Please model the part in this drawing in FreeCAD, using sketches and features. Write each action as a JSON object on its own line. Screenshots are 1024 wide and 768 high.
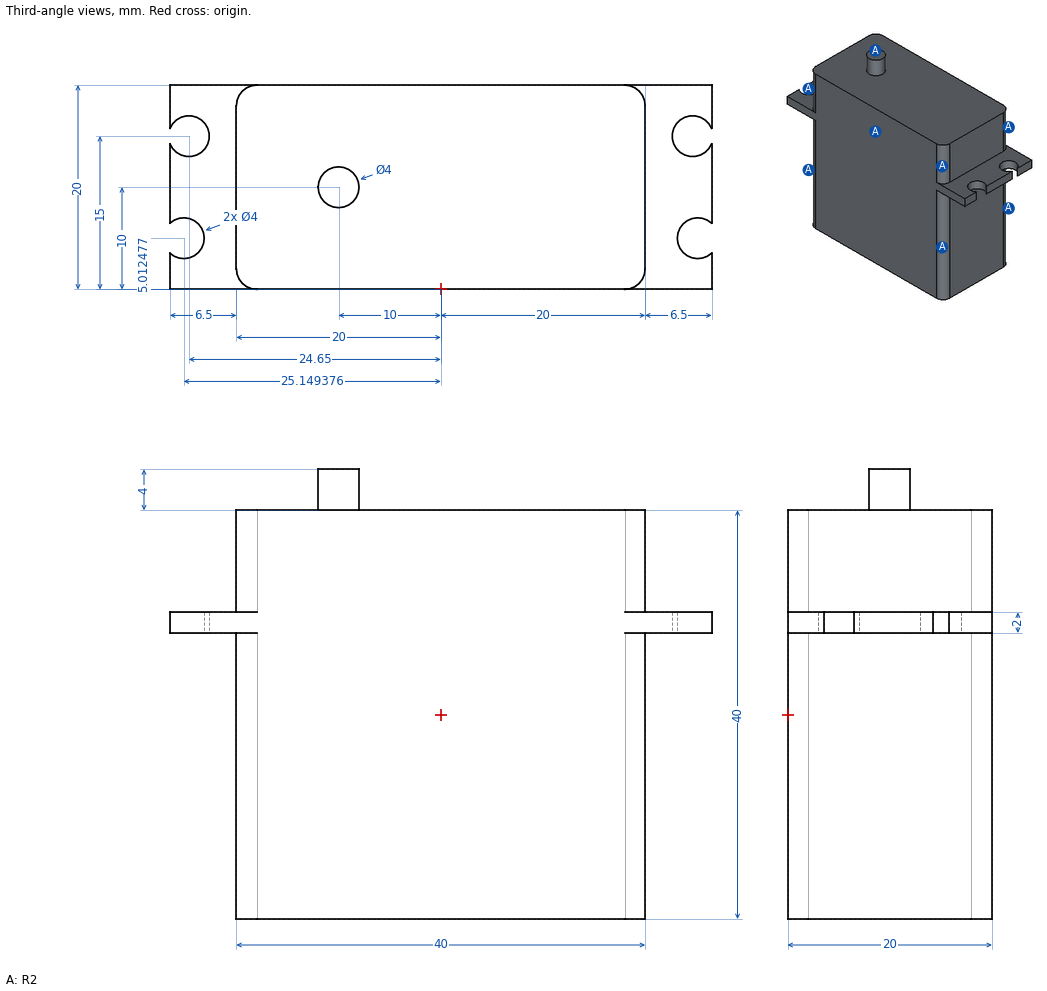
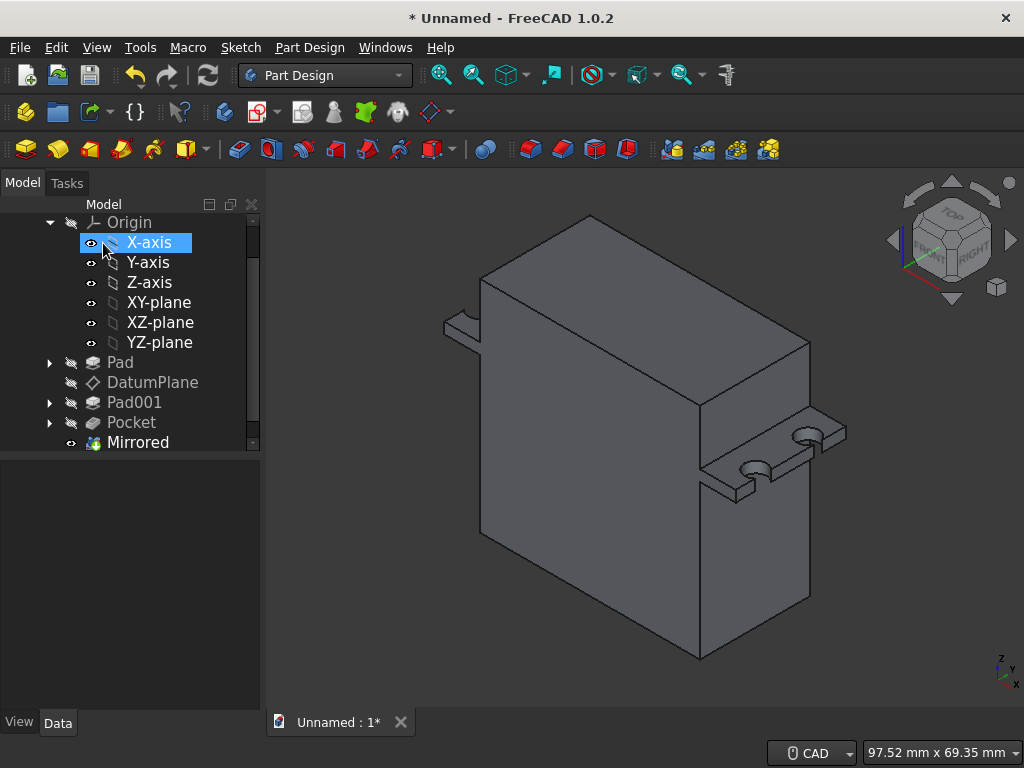
{"action": "left_click", "coordinate": [676, 328]}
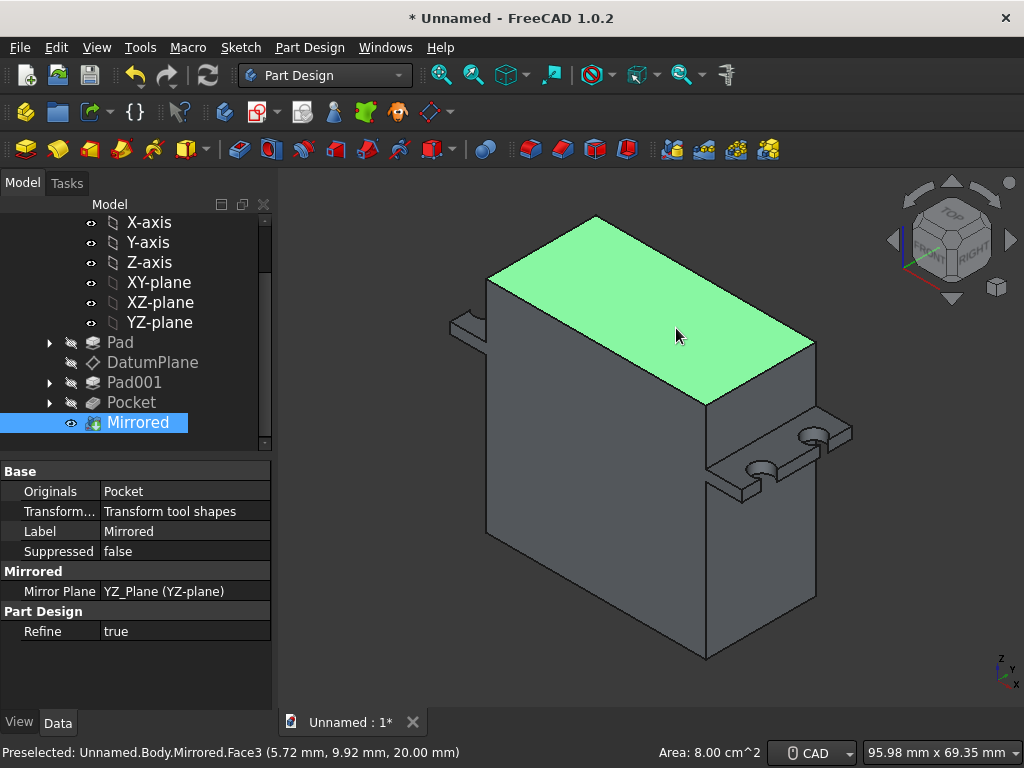
{"action": "left_click", "coordinate": [258, 112]}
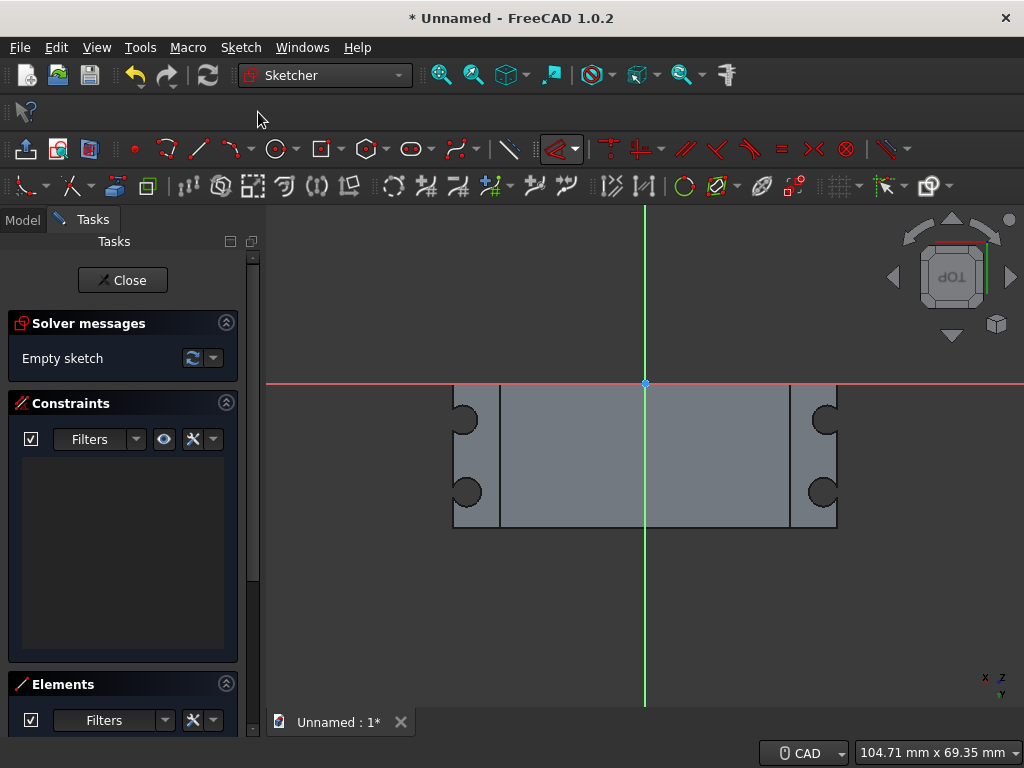
{"action": "scroll", "coordinate": [731, 456], "scroll_direction": "up", "scroll_amount": 12}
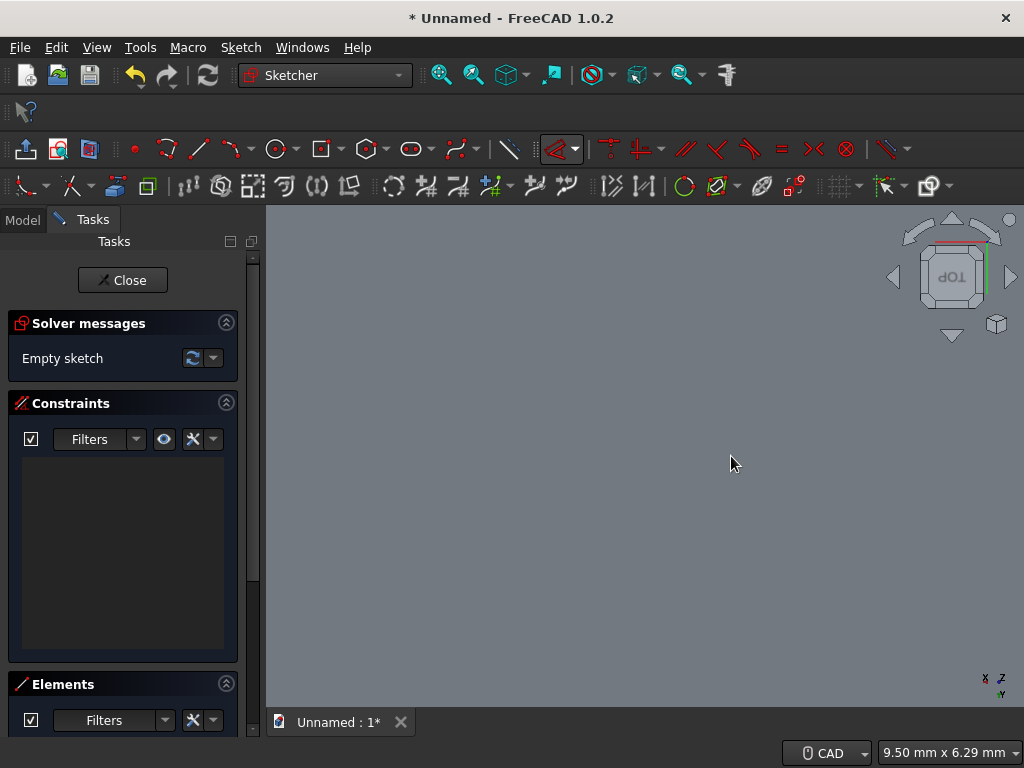
{"action": "left_click", "coordinate": [276, 150]}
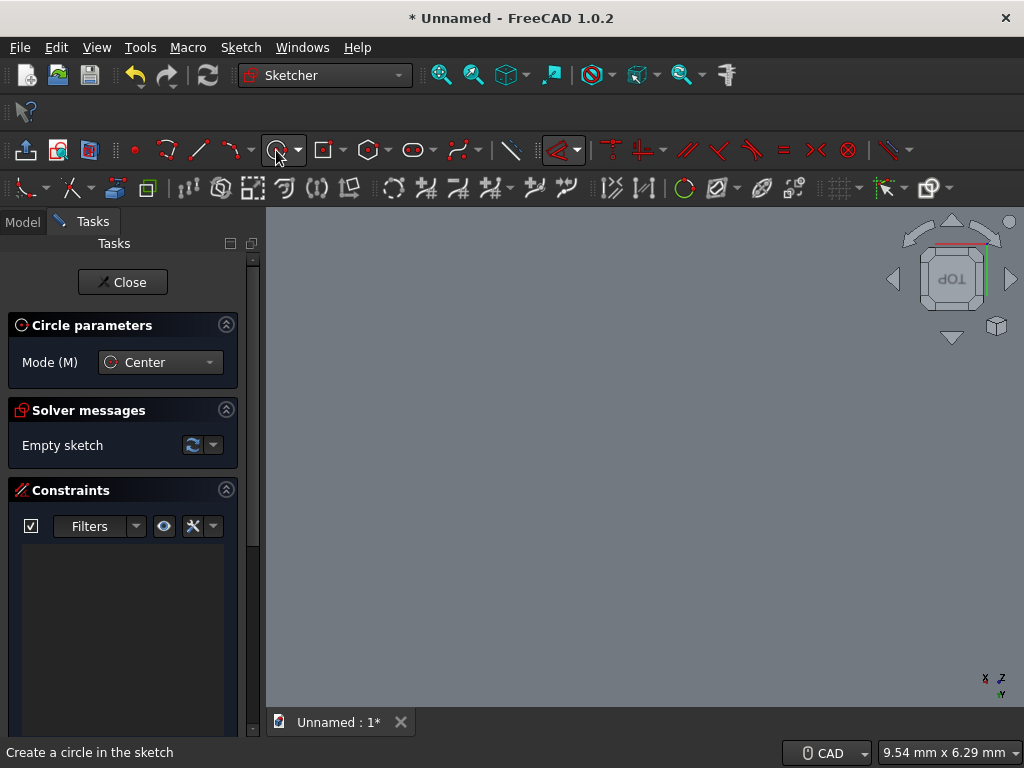
{"action": "left_click", "coordinate": [575, 452]}
{"action": "left_click", "coordinate": [687, 340]}
{"action": "key", "text": "Escape"}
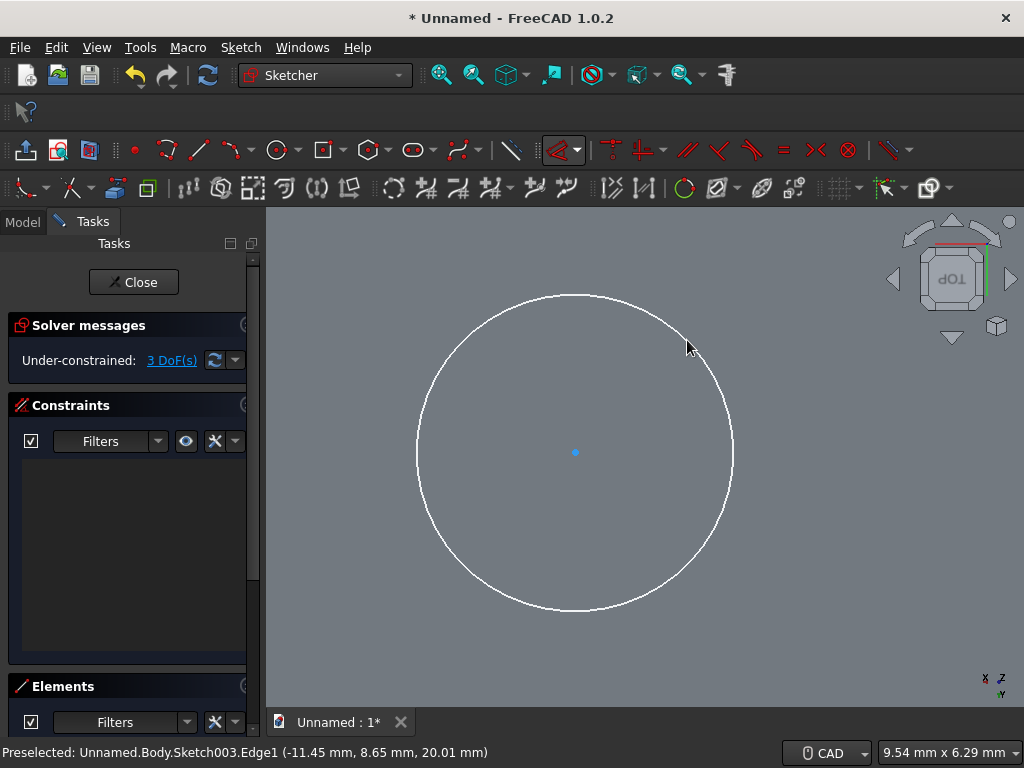
{"action": "left_click", "coordinate": [687, 341]}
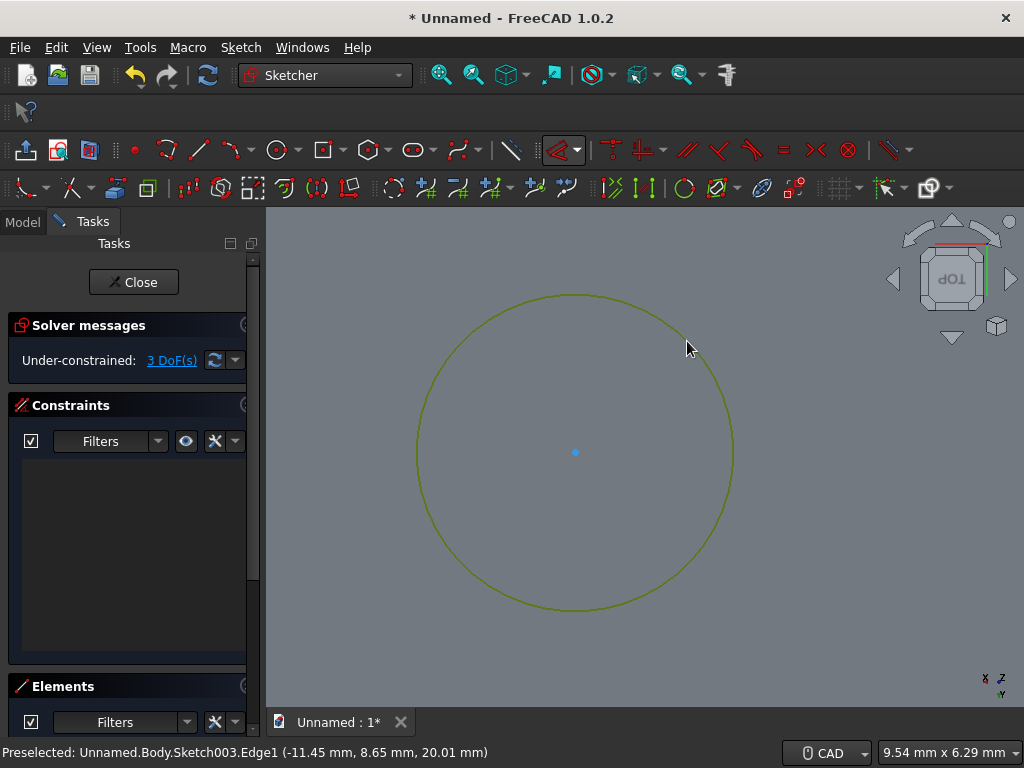
{"action": "key", "text": "k o"}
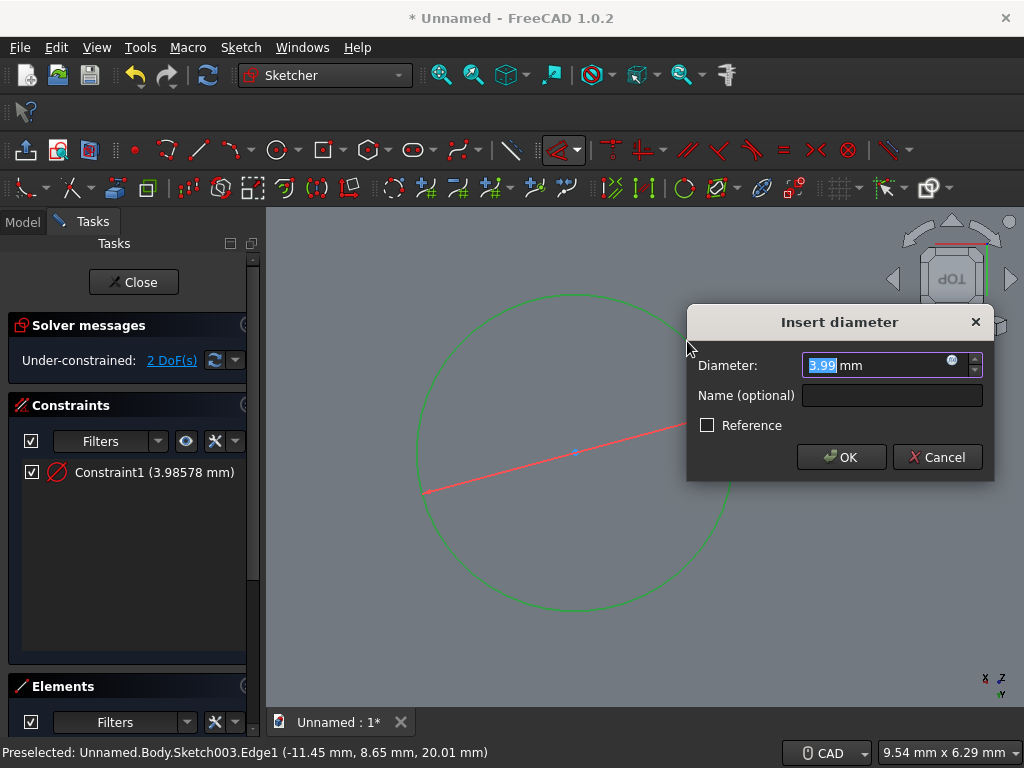
{"action": "type", "text": "4"}
{"action": "key", "text": "Return"}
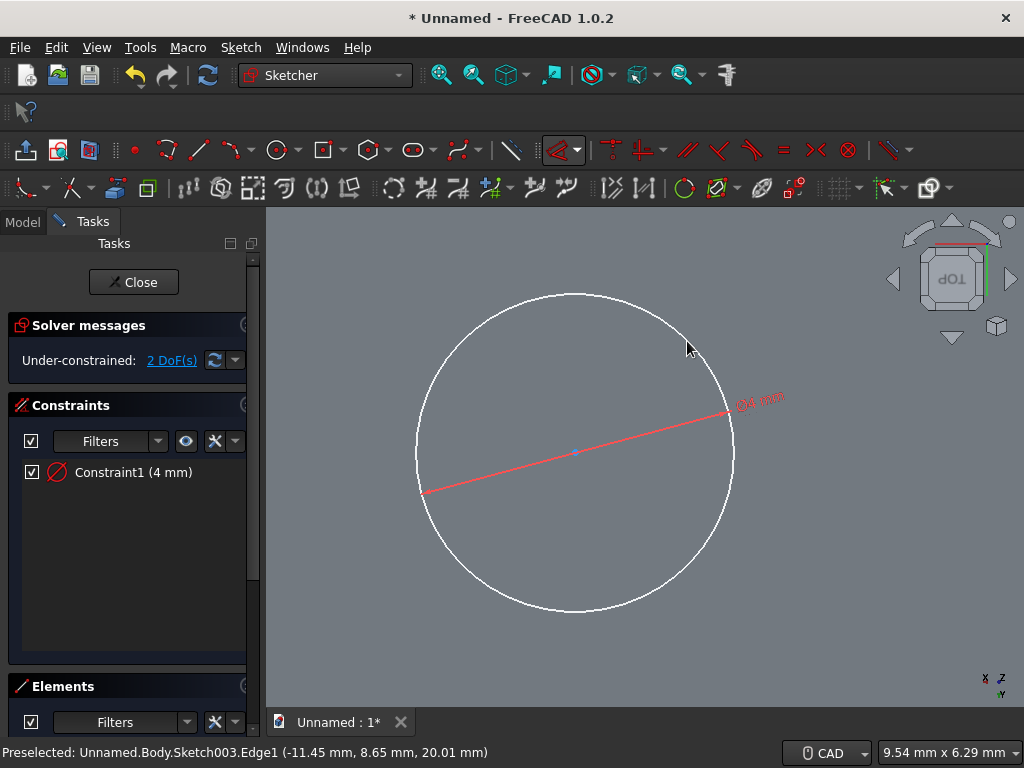
{"action": "left_click", "coordinate": [575, 453]}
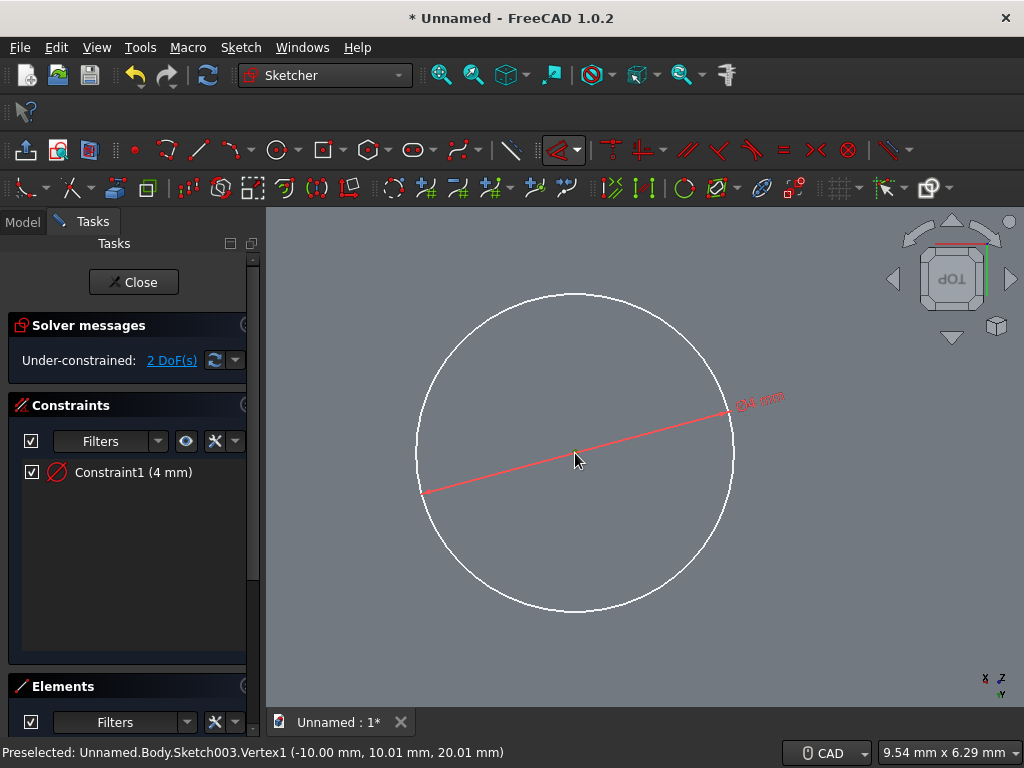
{"action": "key", "text": "l"}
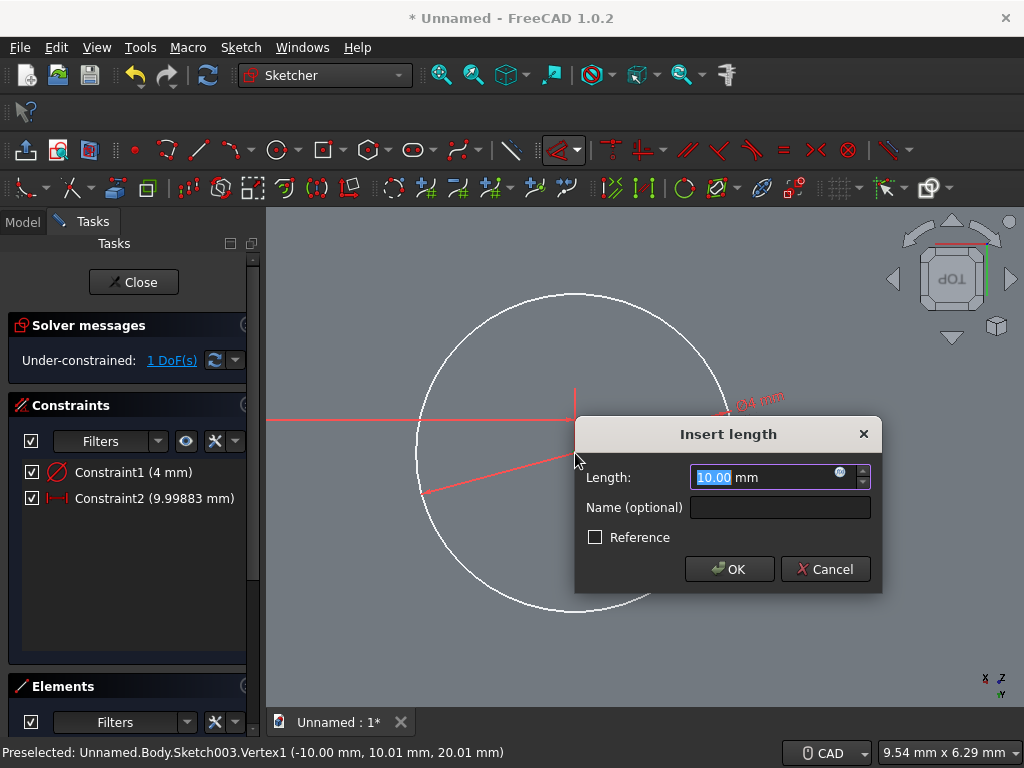
{"action": "type", "text": "10"}
{"action": "key", "text": "Return"}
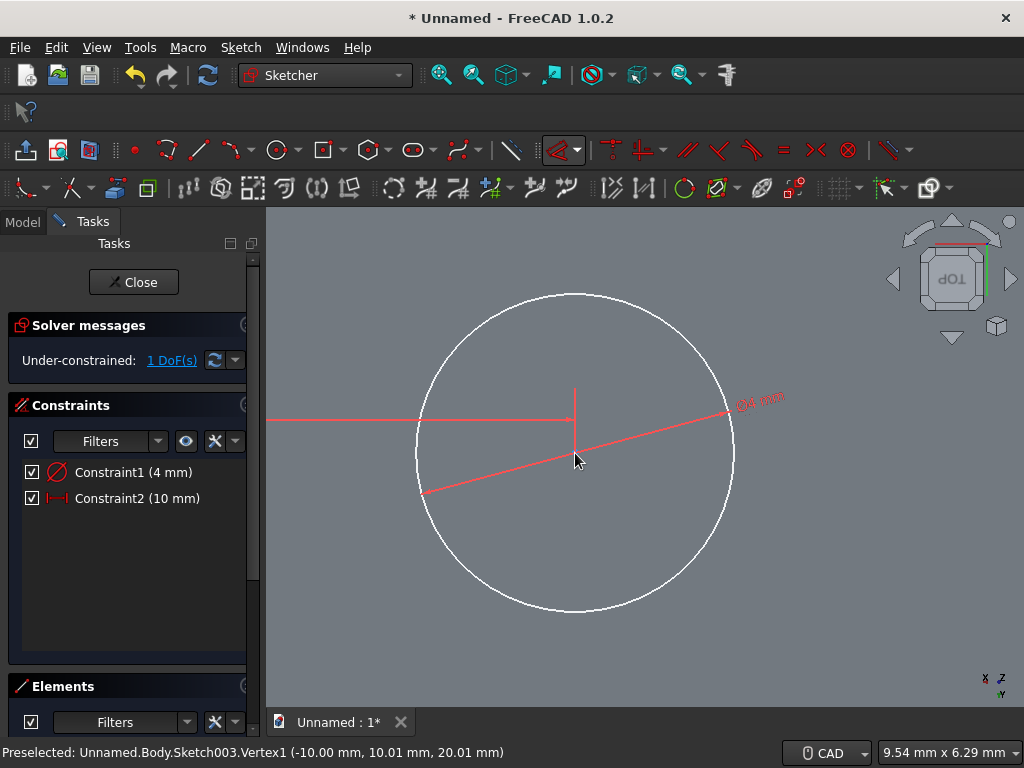
{"action": "left_click", "coordinate": [575, 453]}